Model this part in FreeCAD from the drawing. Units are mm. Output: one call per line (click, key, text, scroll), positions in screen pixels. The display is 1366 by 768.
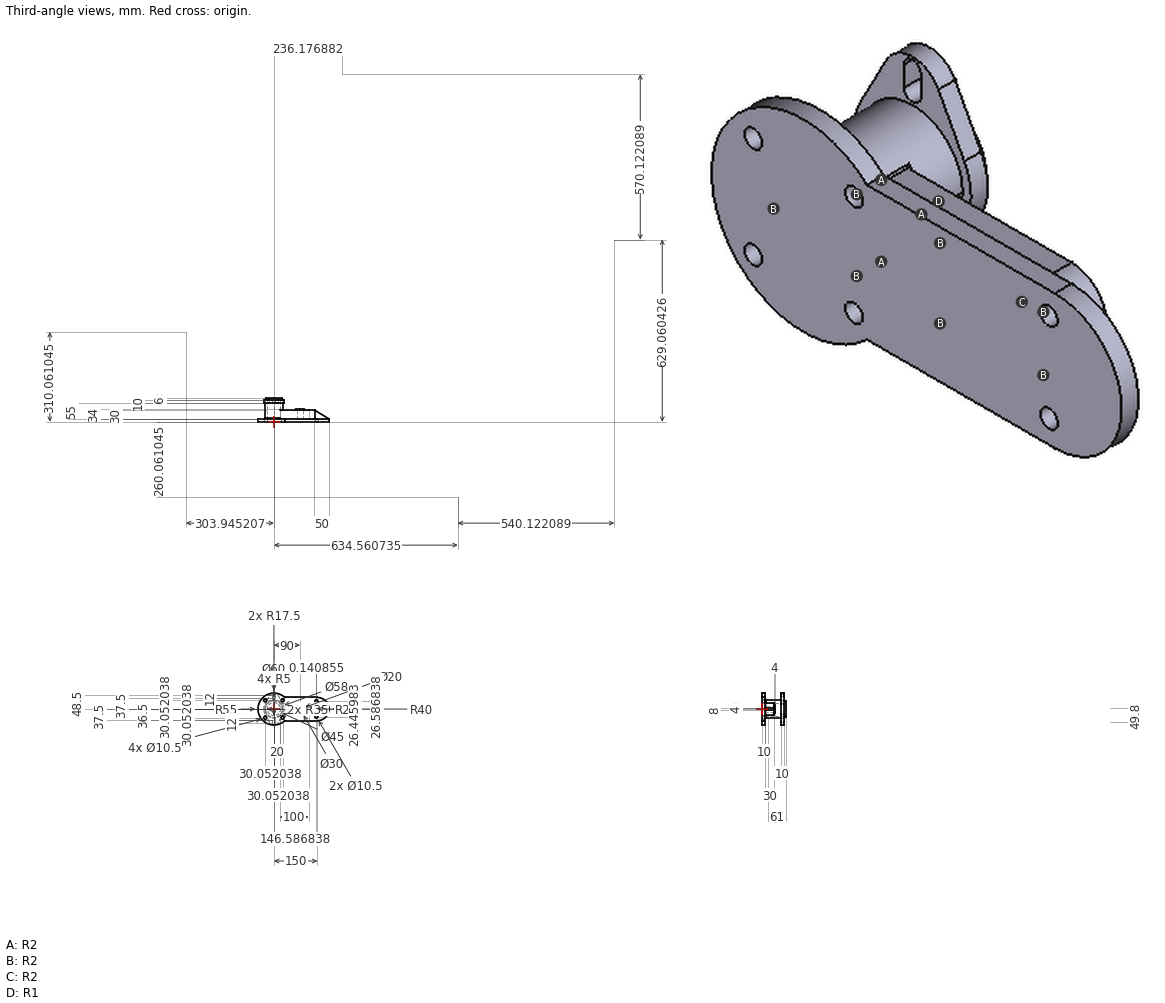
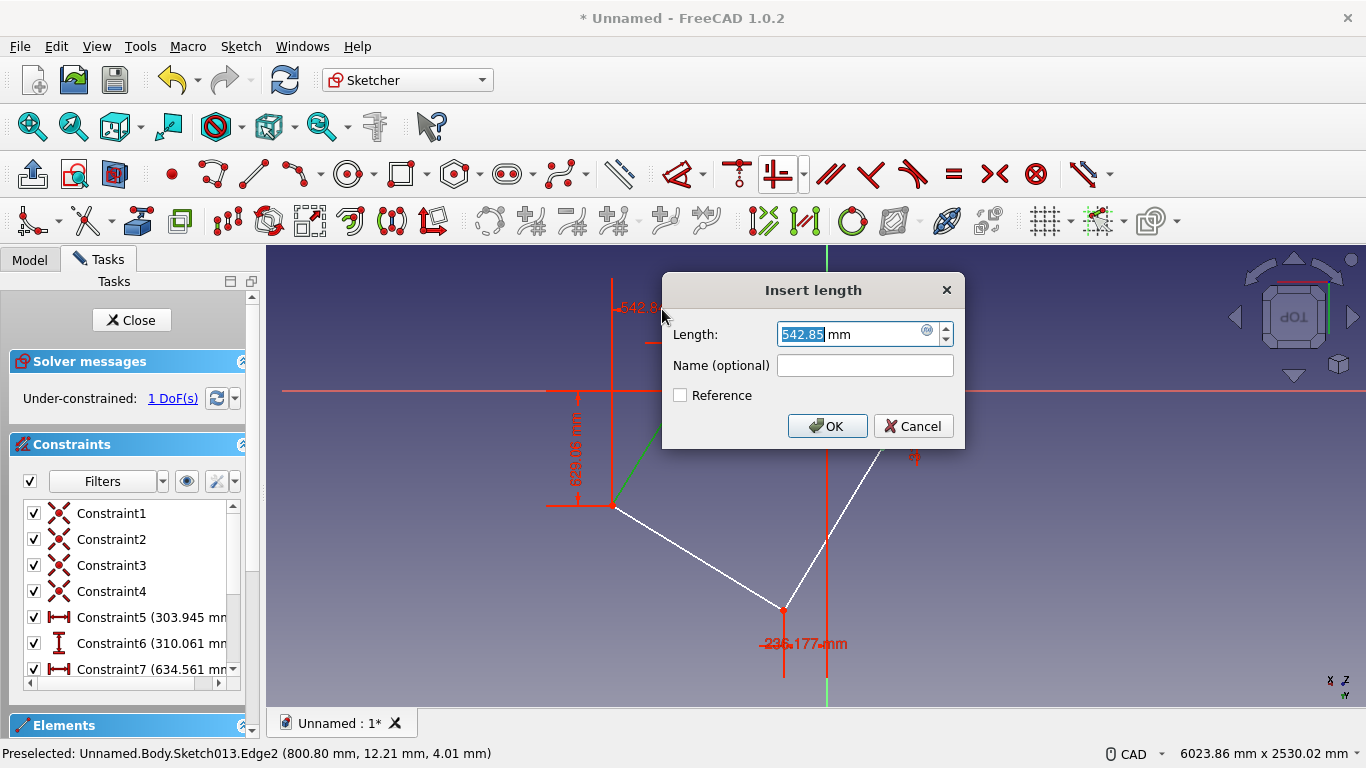
text(540.122089)
key(Return)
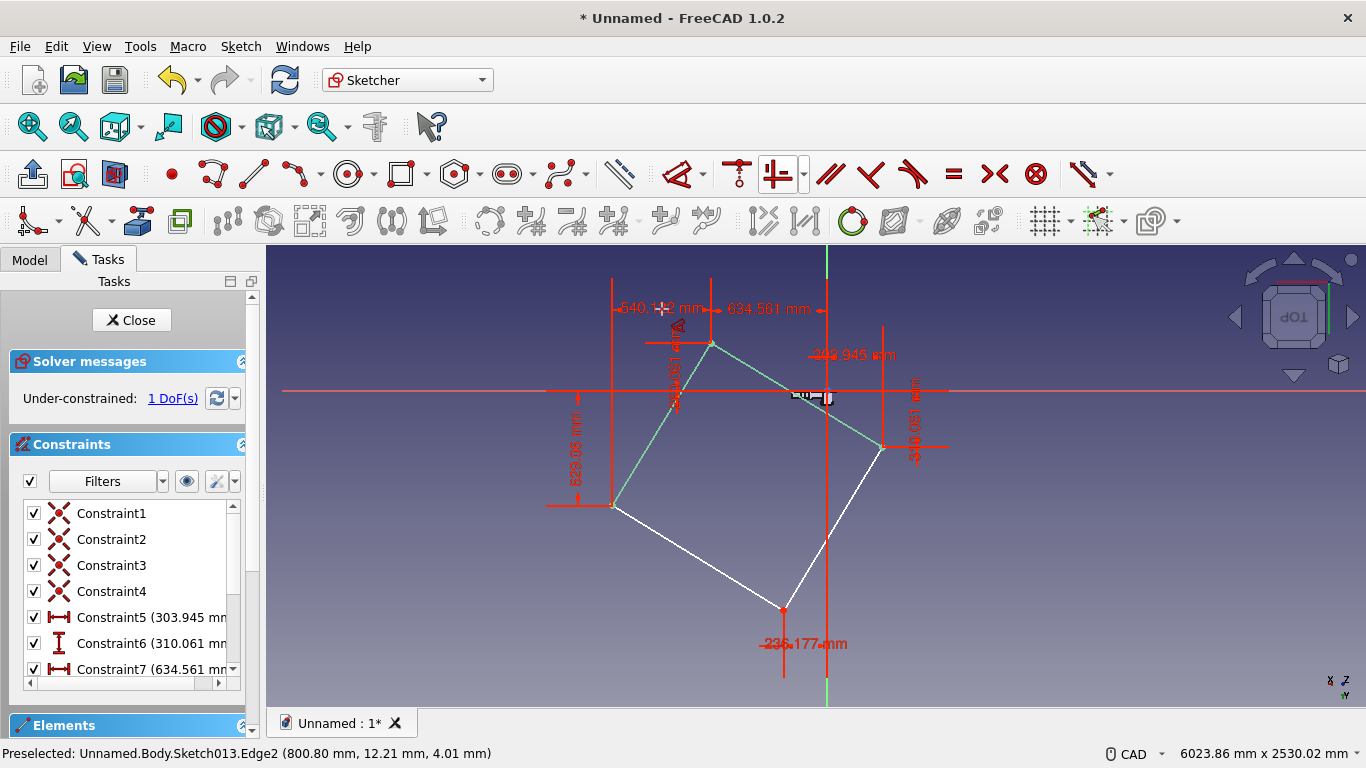
click(664, 537)
click(578, 558)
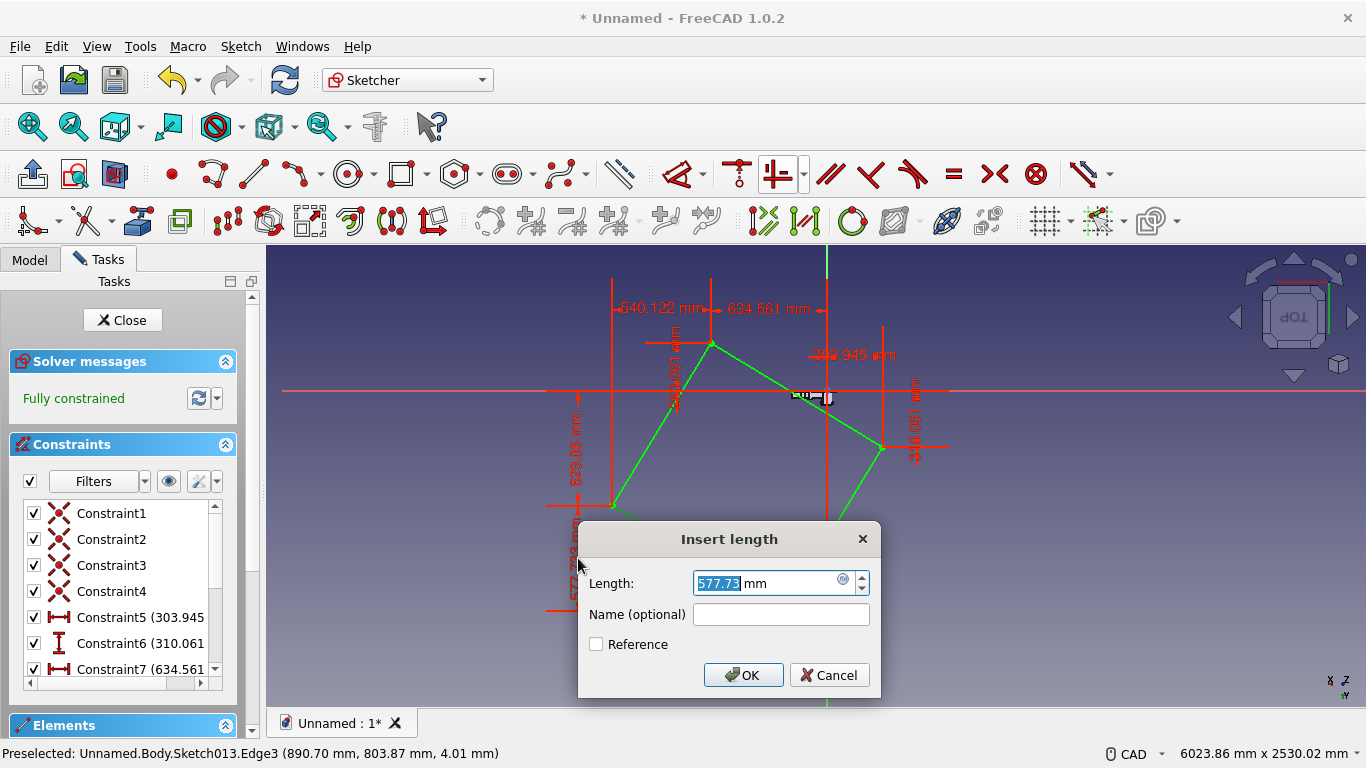
text(570.122089)
key(Return)
key(Escape)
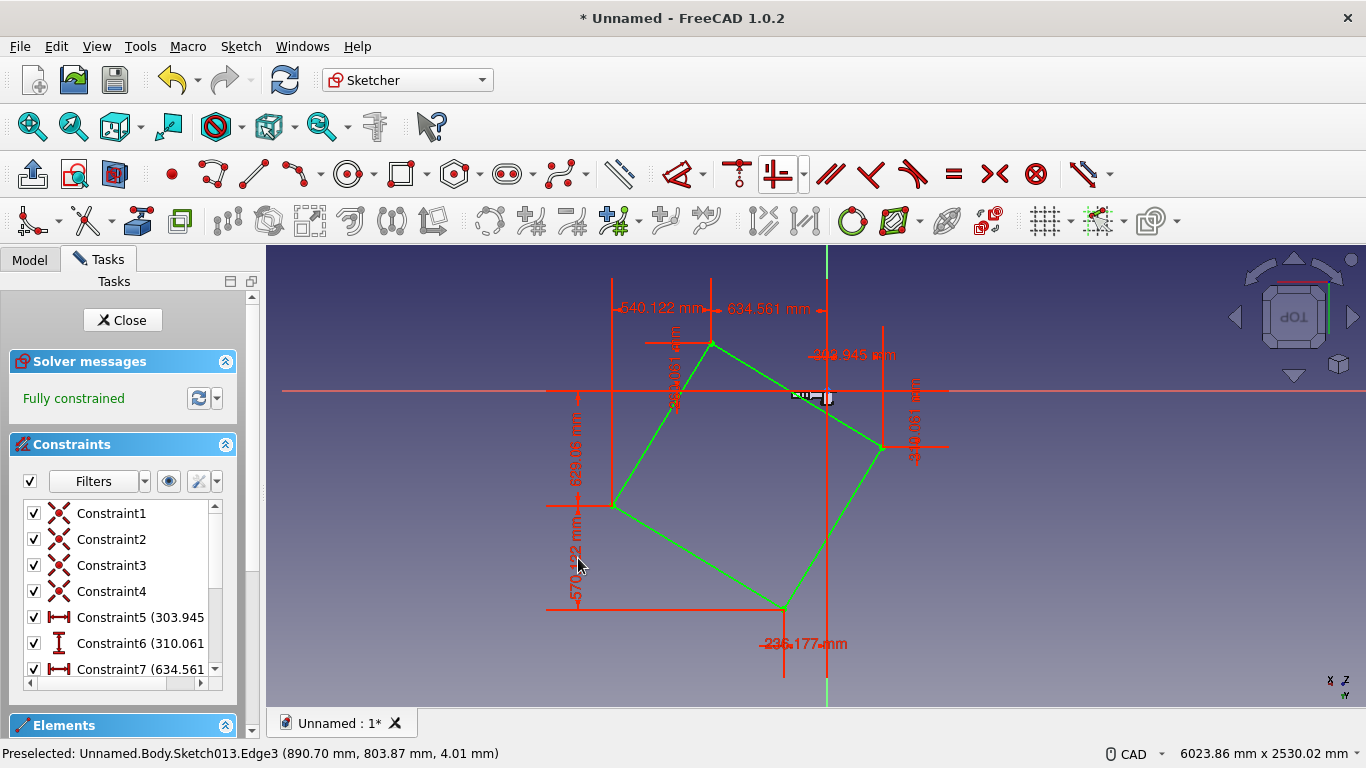
click(123, 320)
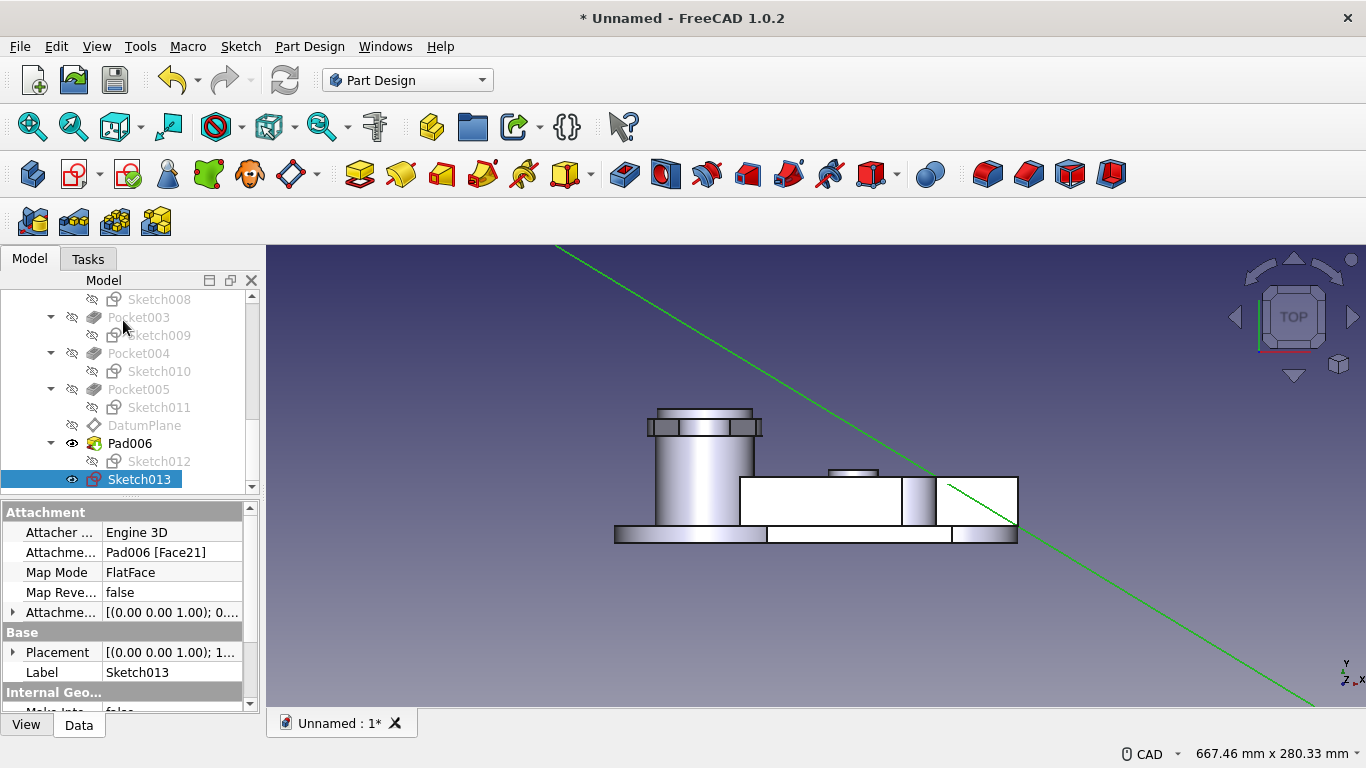
click(625, 174)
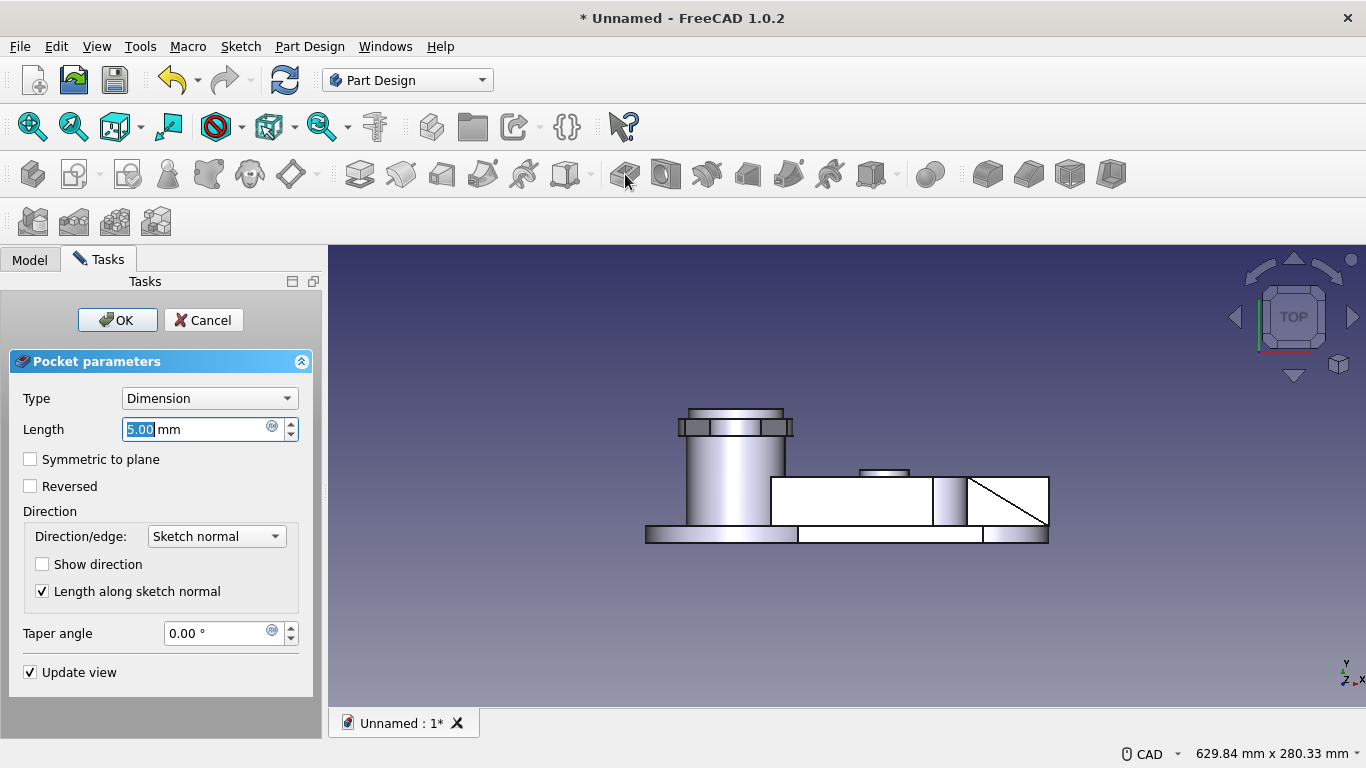
click(210, 398)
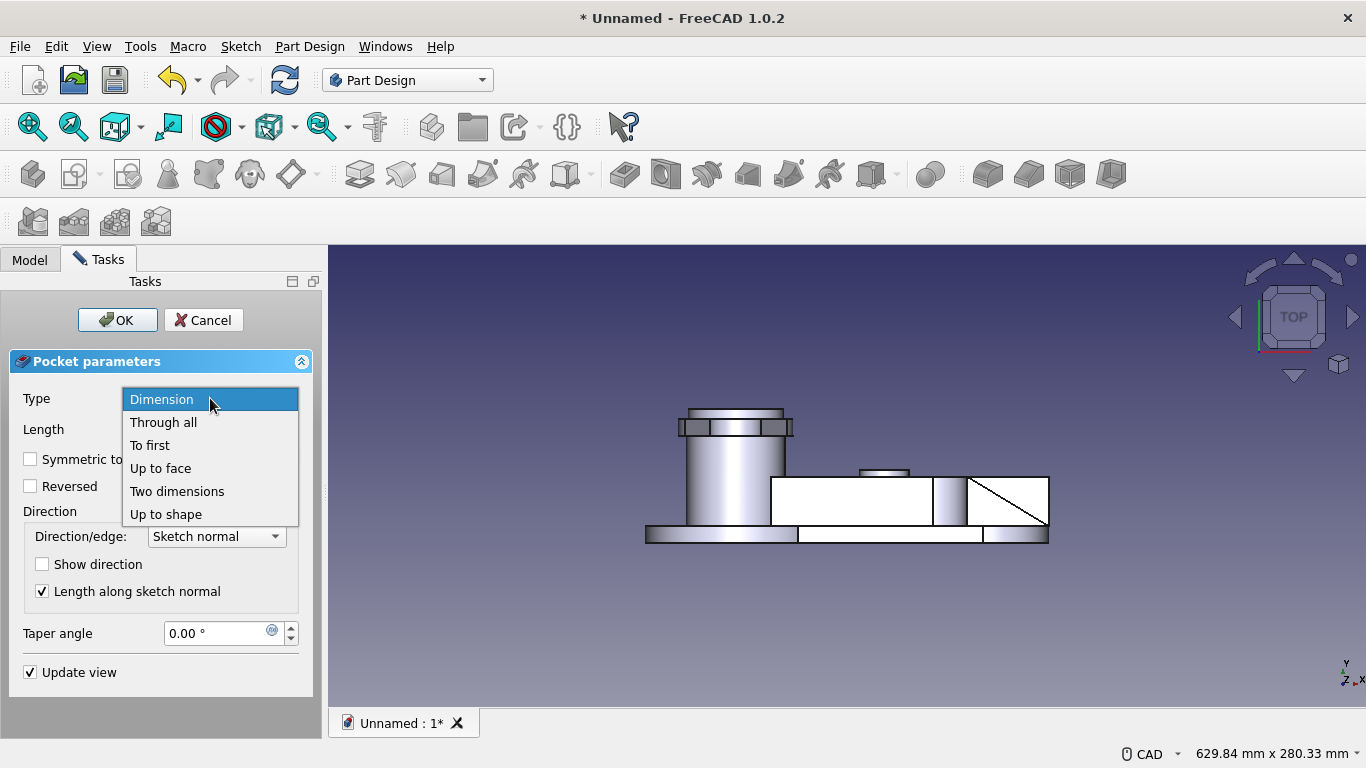
click(208, 492)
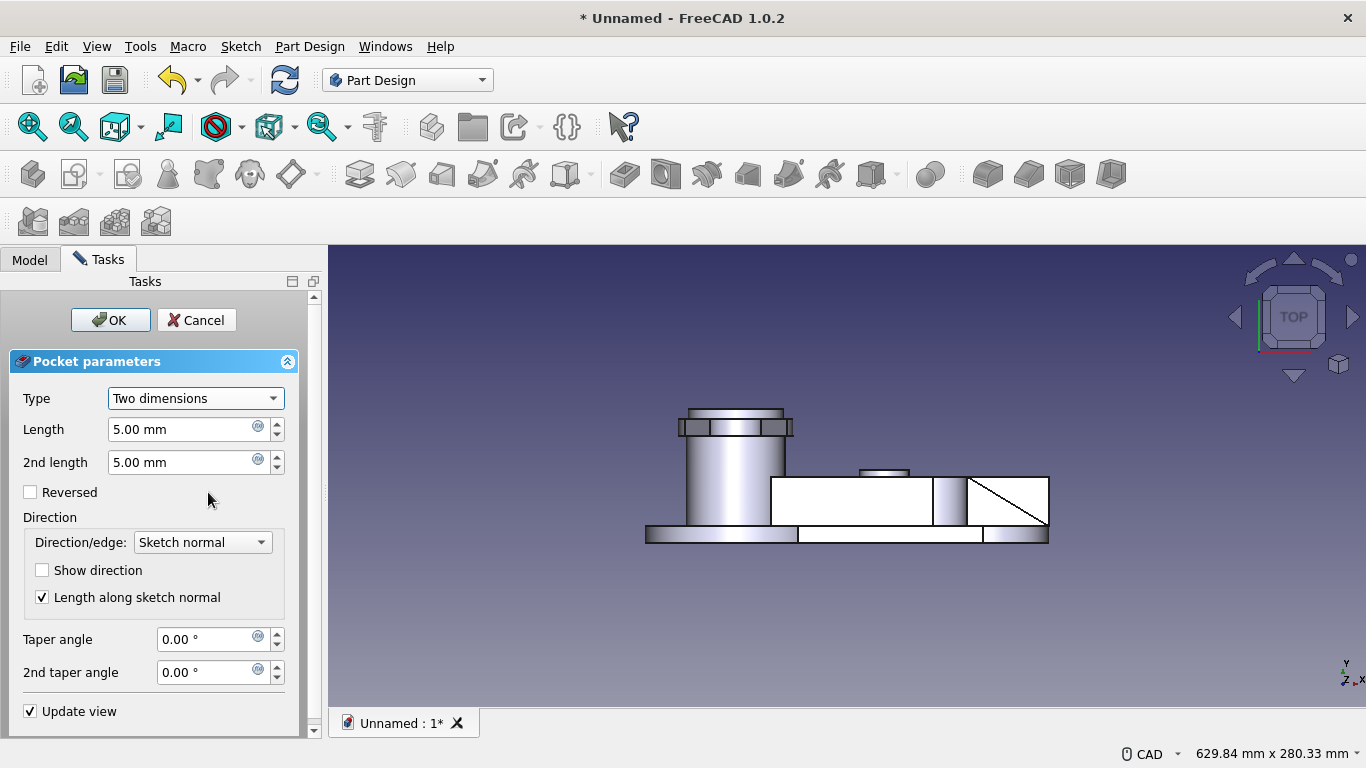
triple_click(190, 430)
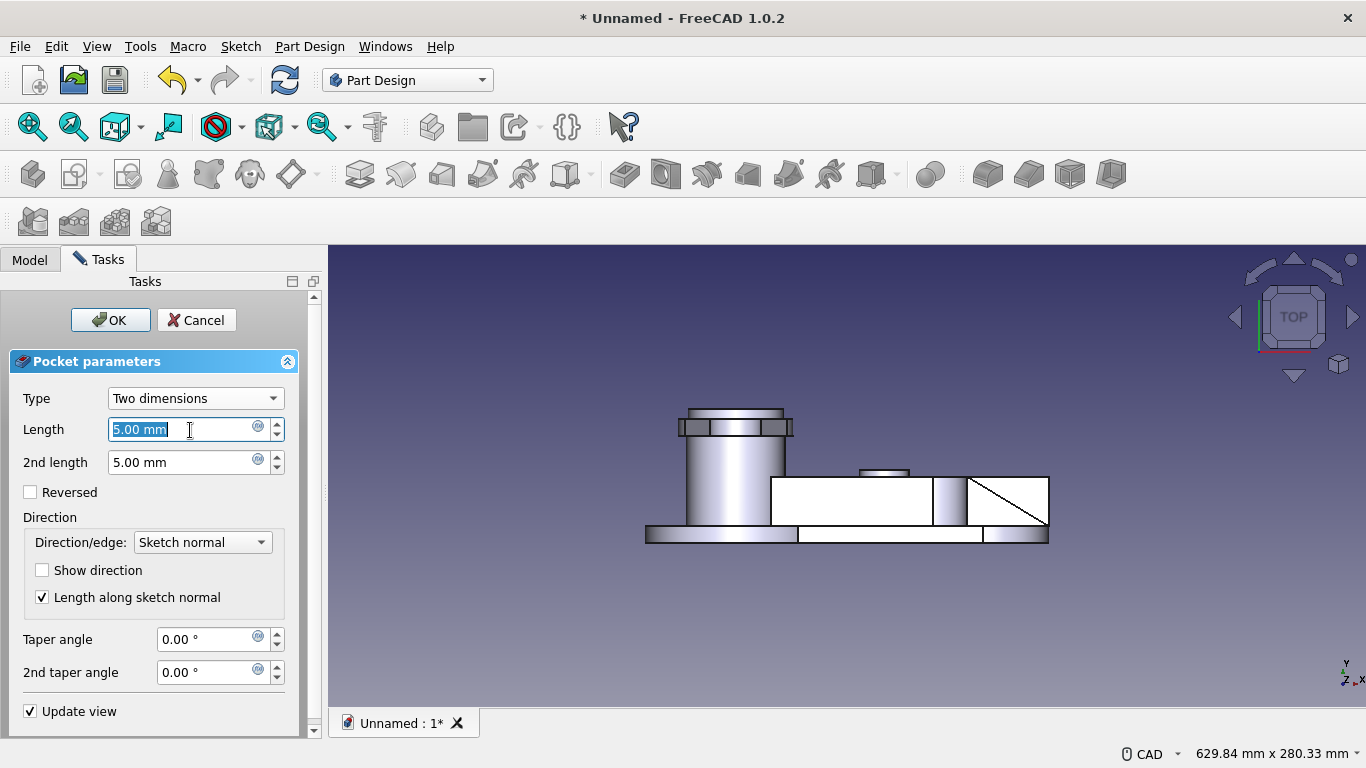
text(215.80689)
key(Tab)